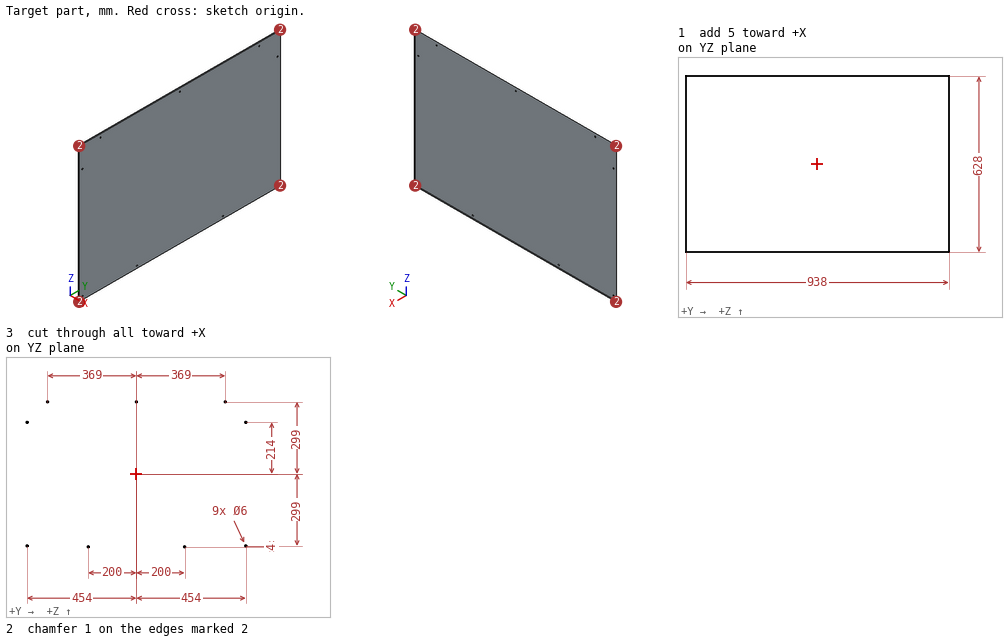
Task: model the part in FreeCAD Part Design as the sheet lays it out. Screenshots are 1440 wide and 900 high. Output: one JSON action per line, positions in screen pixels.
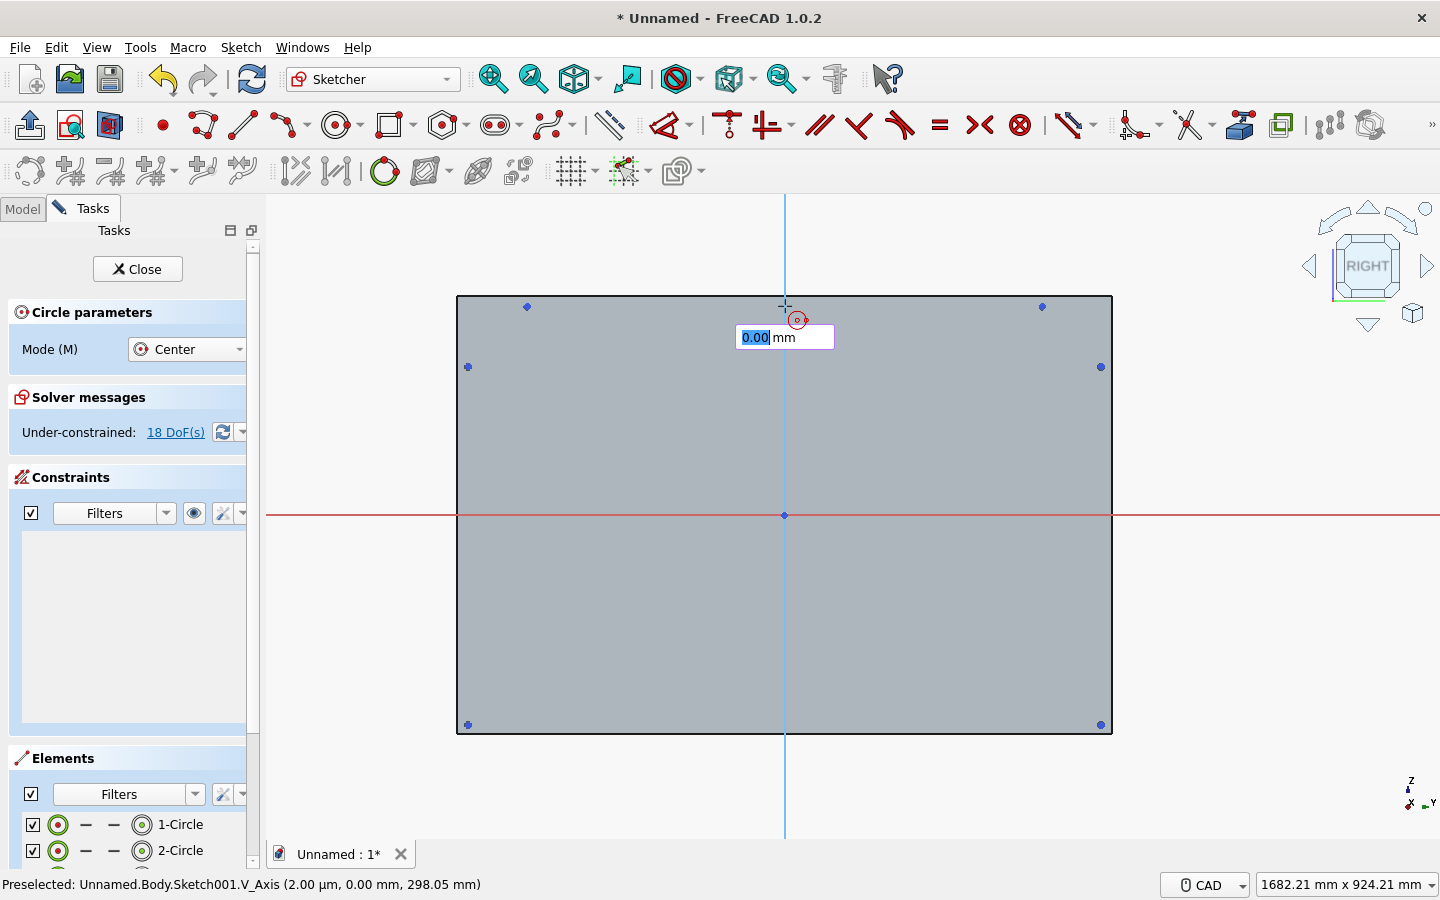
{"action": "scroll", "coordinate": [787, 306], "scroll_direction": "up", "scroll_amount": 11}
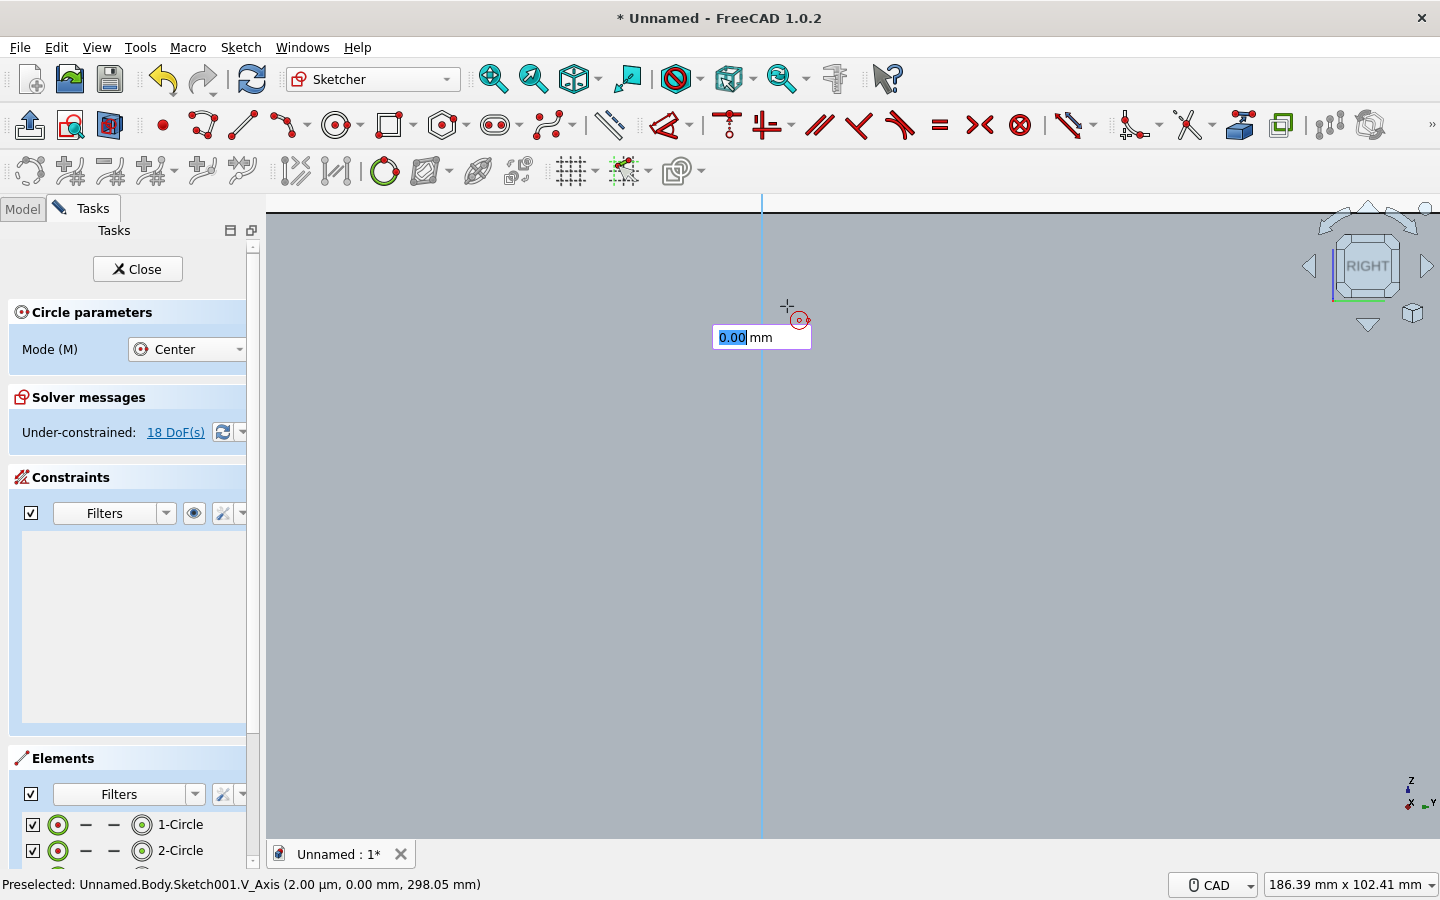
{"action": "left_click", "coordinate": [779, 301]}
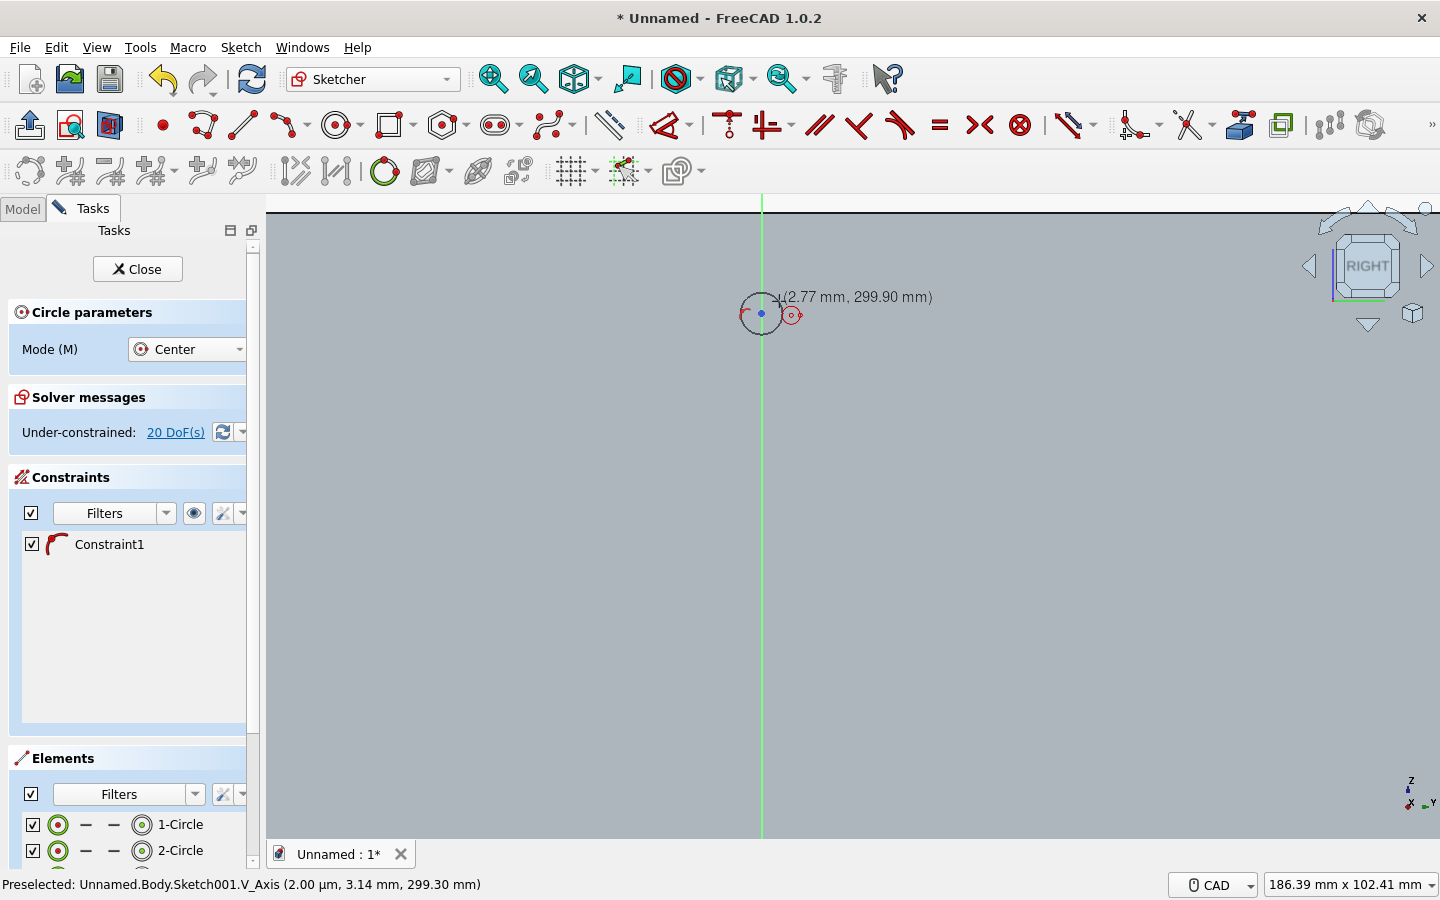
{"action": "scroll", "coordinate": [787, 306], "scroll_direction": "down", "scroll_amount": 11}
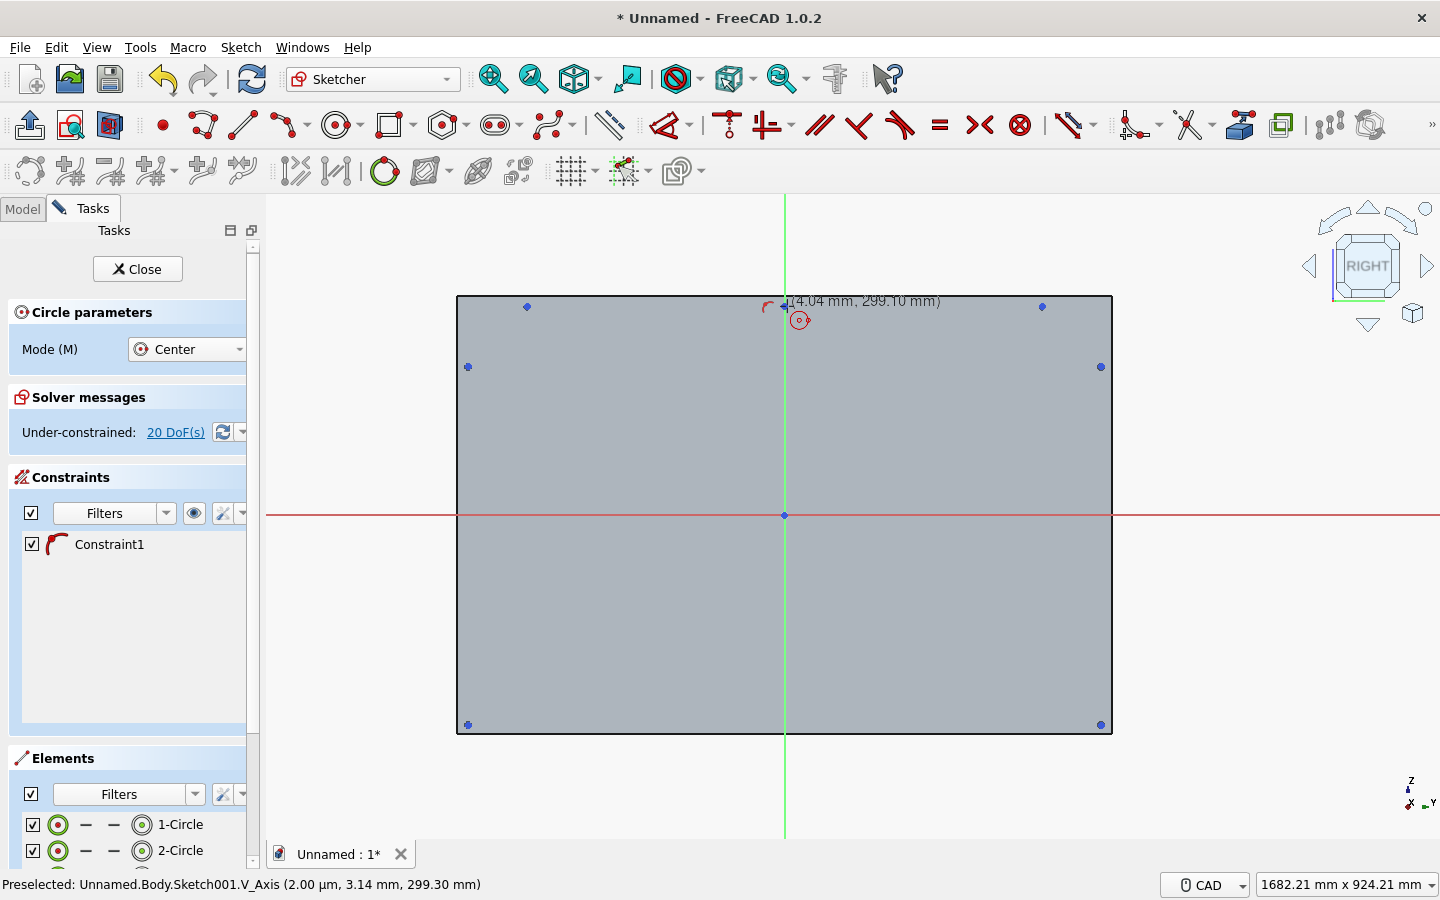
{"action": "scroll", "coordinate": [924, 726], "scroll_direction": "up", "scroll_amount": 12}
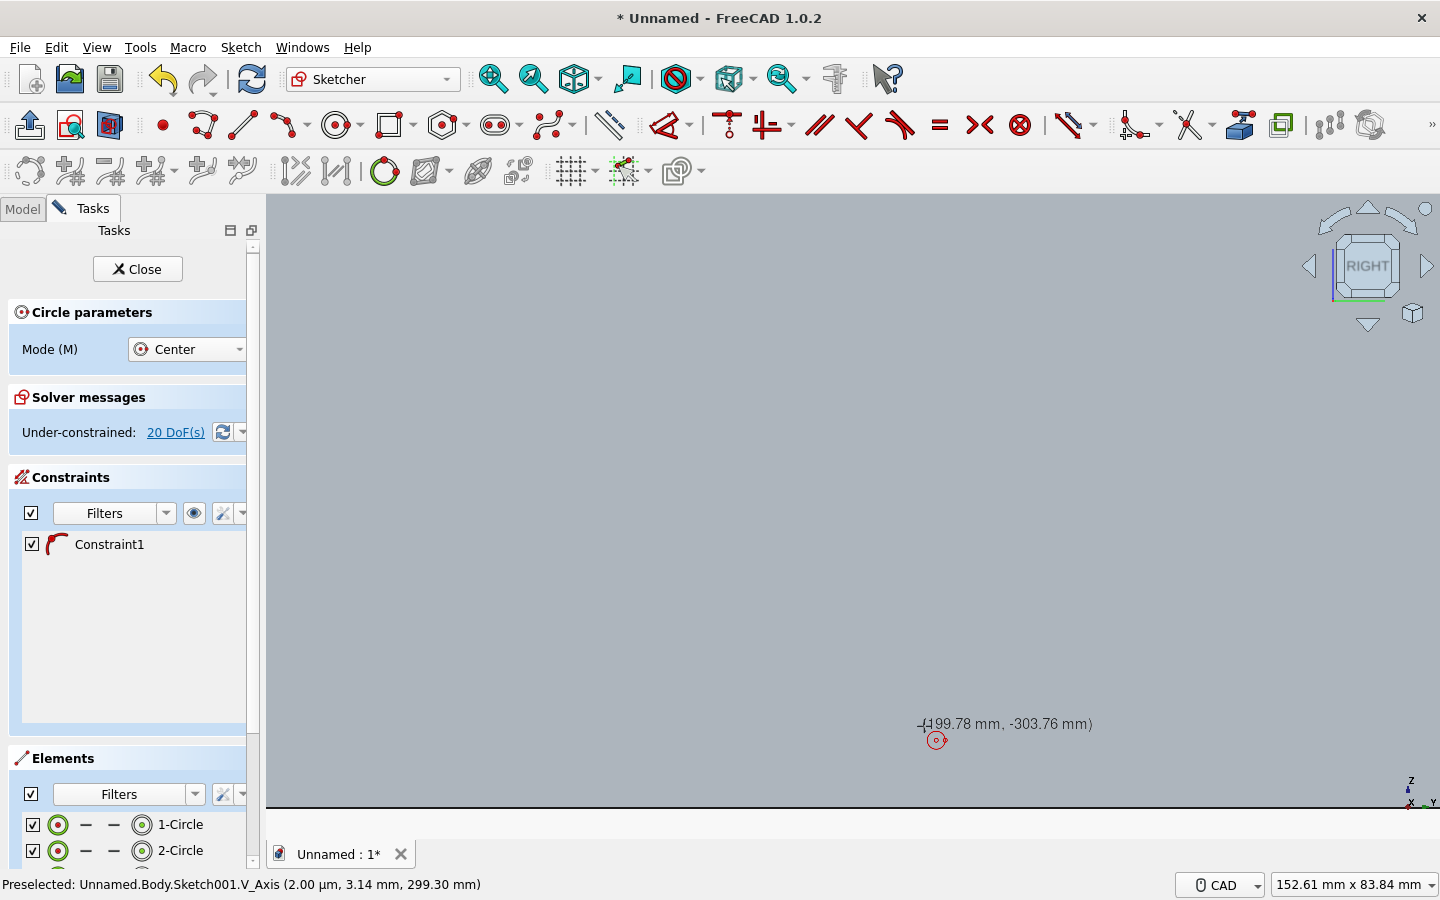
{"action": "scroll", "coordinate": [924, 727], "scroll_direction": "down", "scroll_amount": 12}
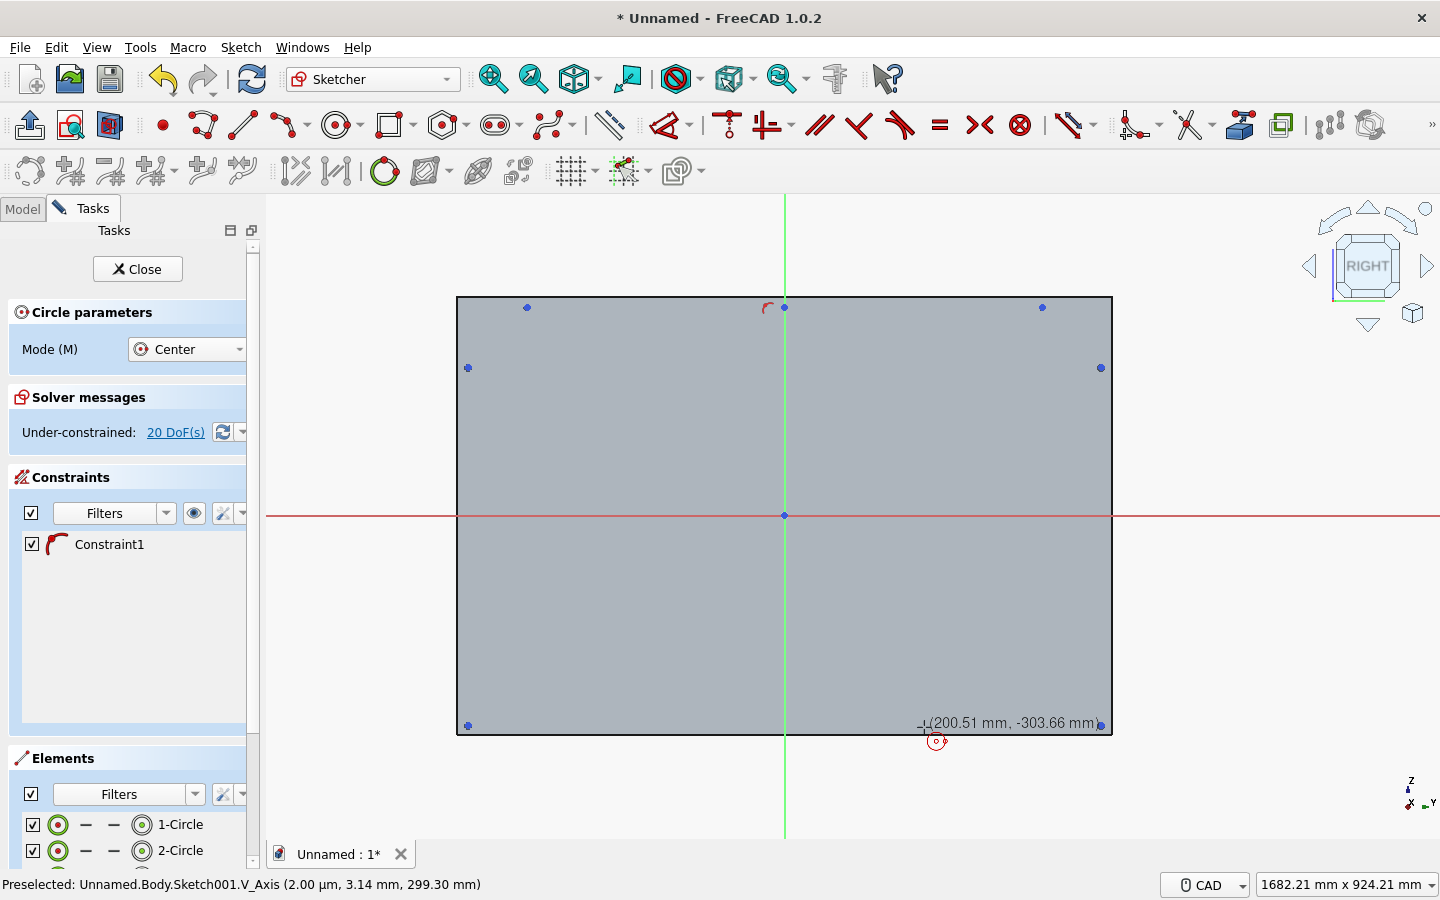
{"action": "left_click", "coordinate": [924, 727]}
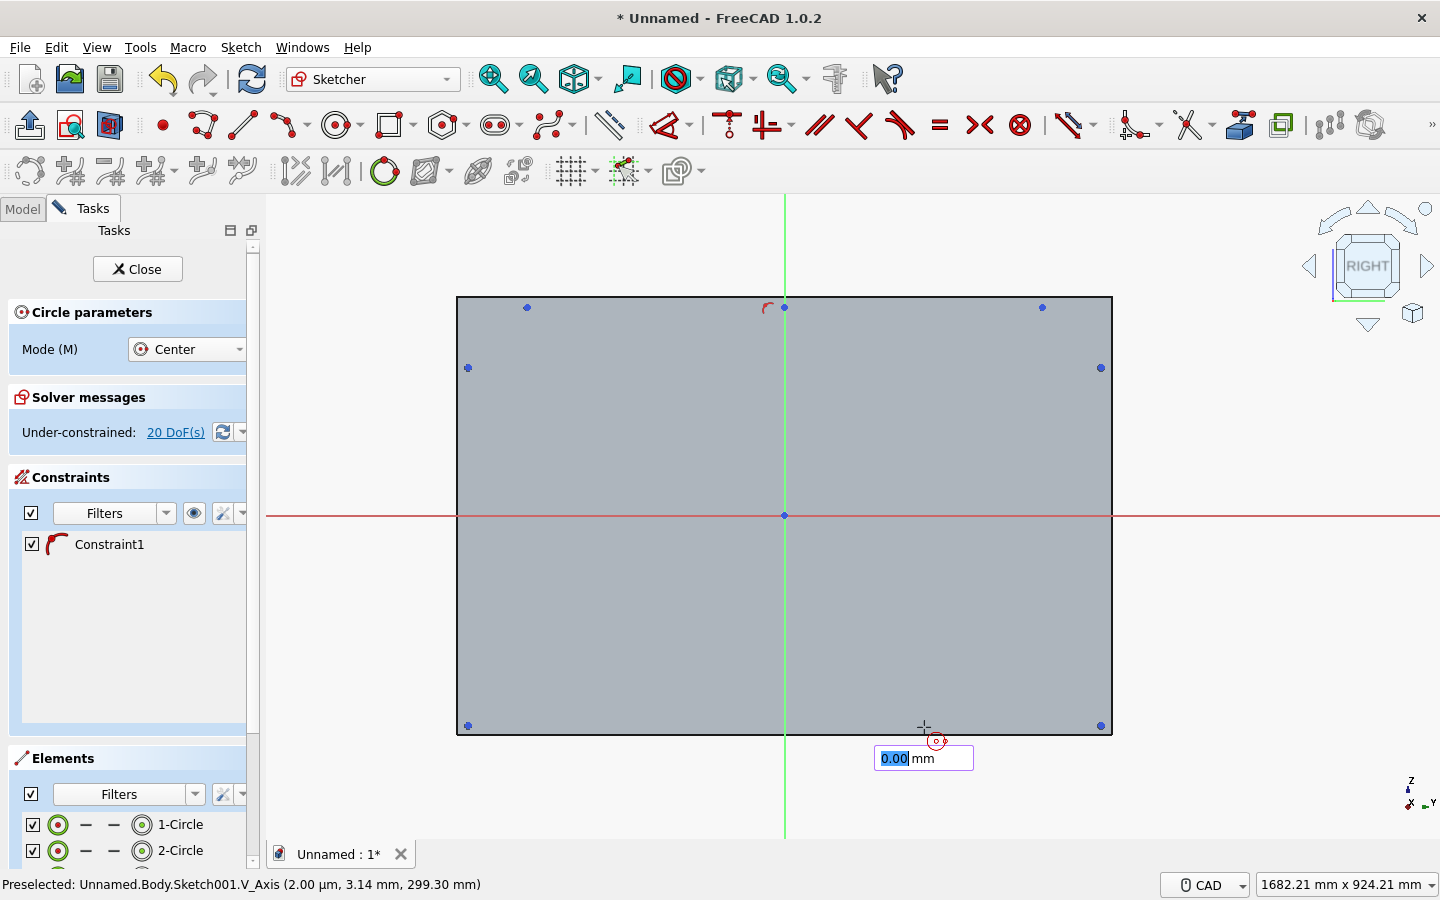
{"action": "scroll", "coordinate": [926, 726], "scroll_direction": "up", "scroll_amount": 11}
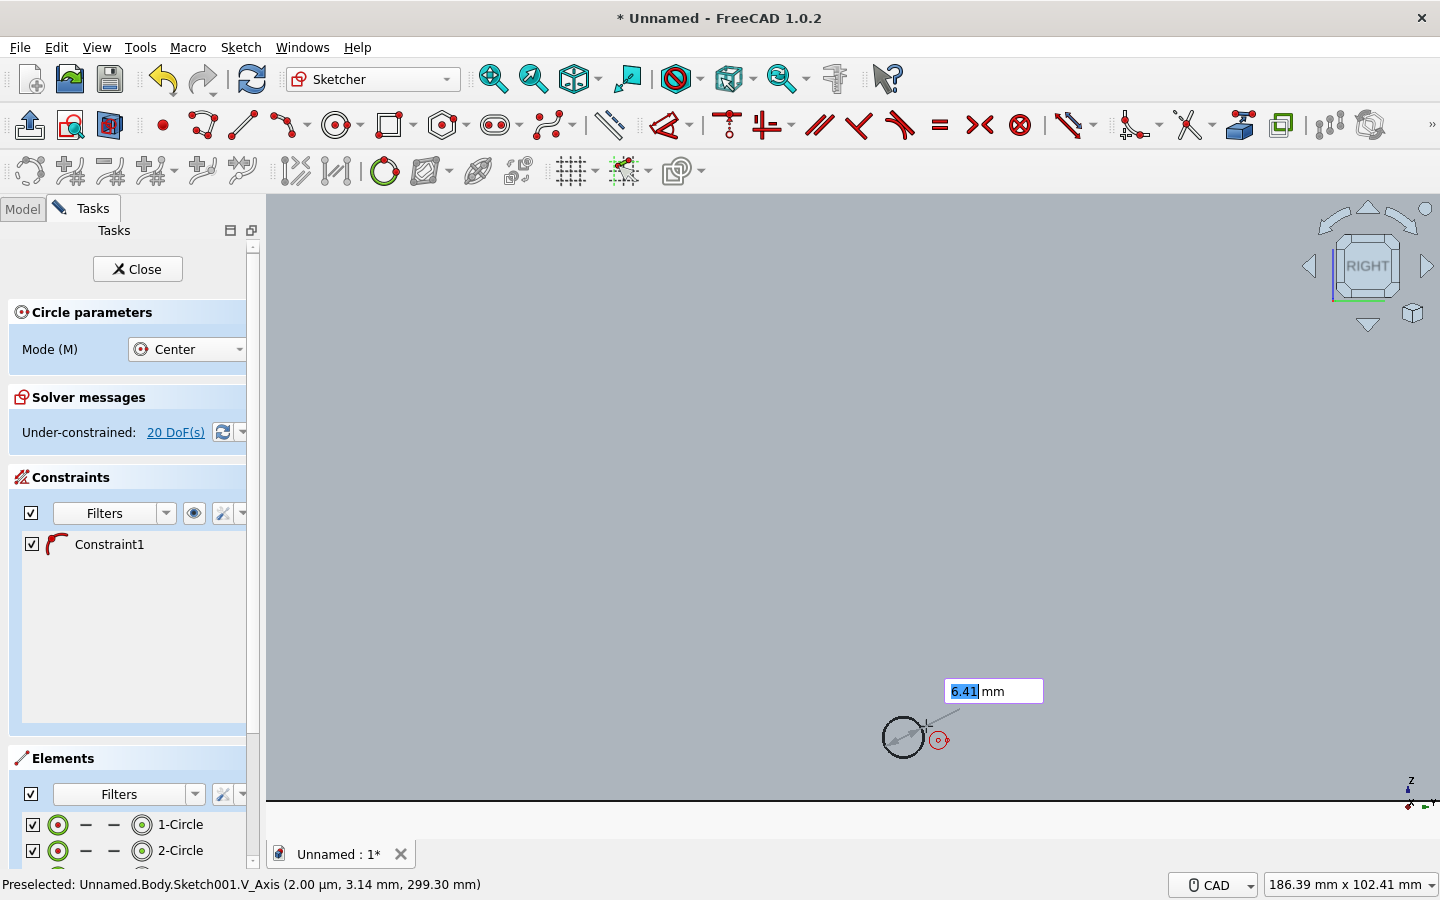
{"action": "left_click", "coordinate": [918, 718]}